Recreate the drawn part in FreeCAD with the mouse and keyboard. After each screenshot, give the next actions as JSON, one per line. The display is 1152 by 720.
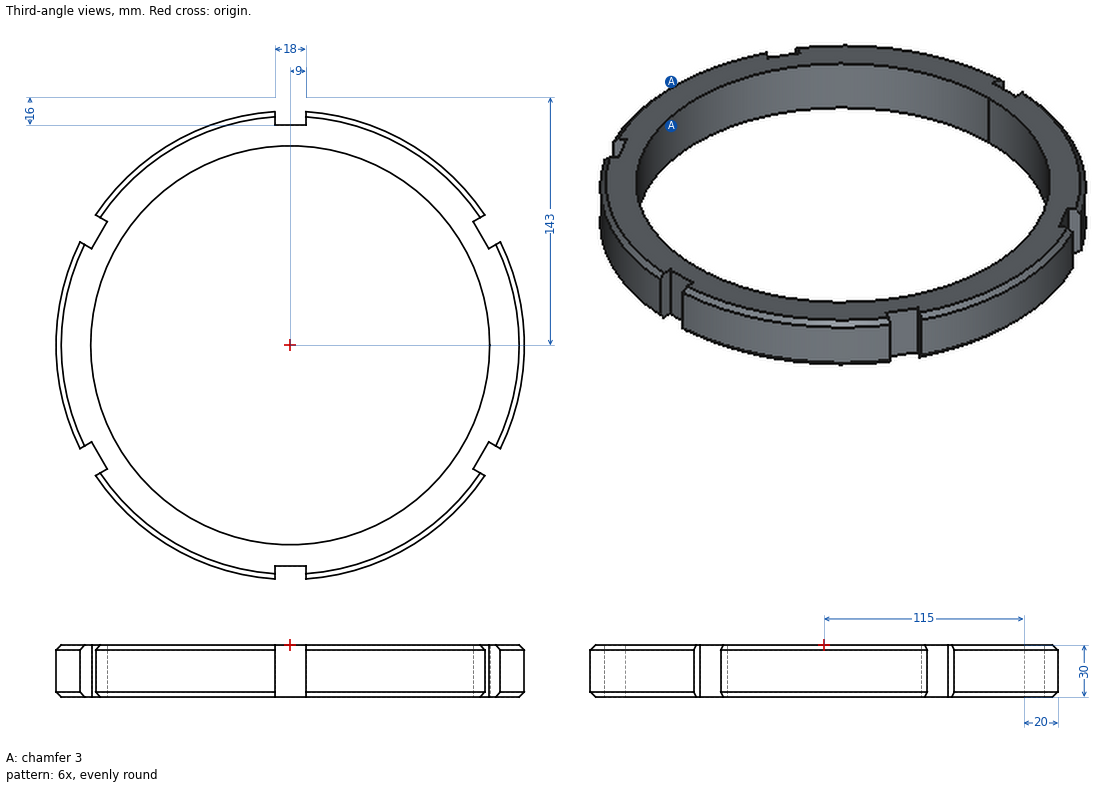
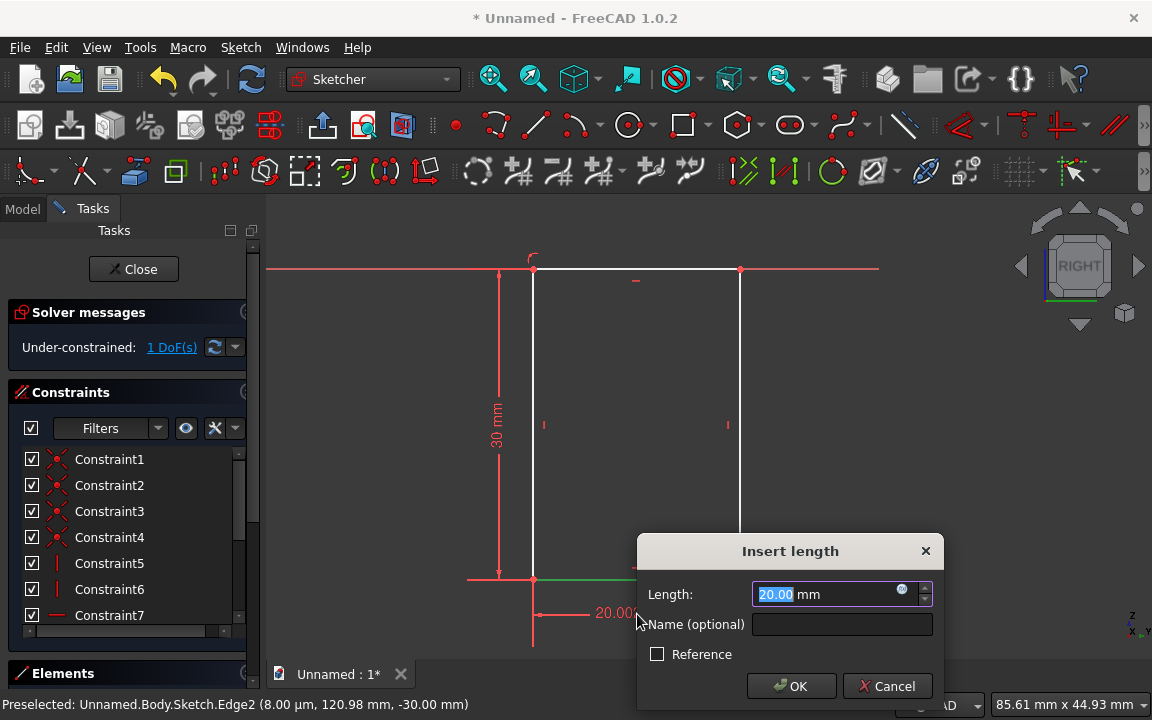
{"action": "type", "text": "20"}
{"action": "key", "text": "Return"}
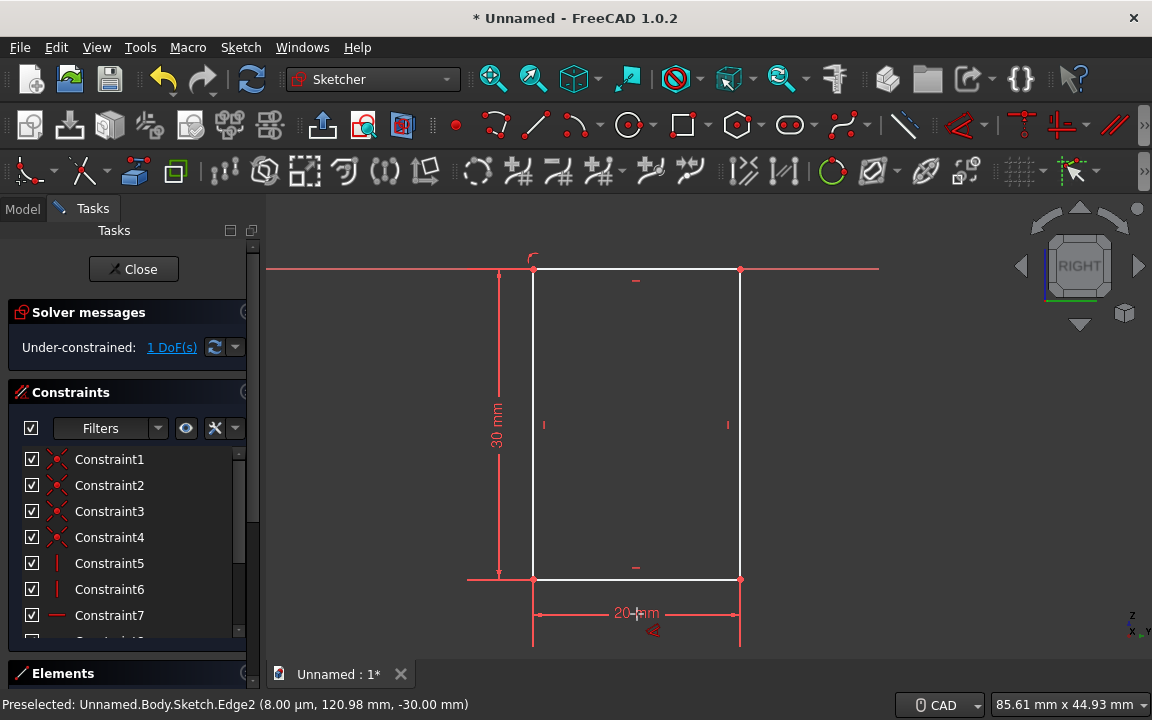
{"action": "left_click", "coordinate": [533, 269]}
{"action": "left_click", "coordinate": [414, 235]}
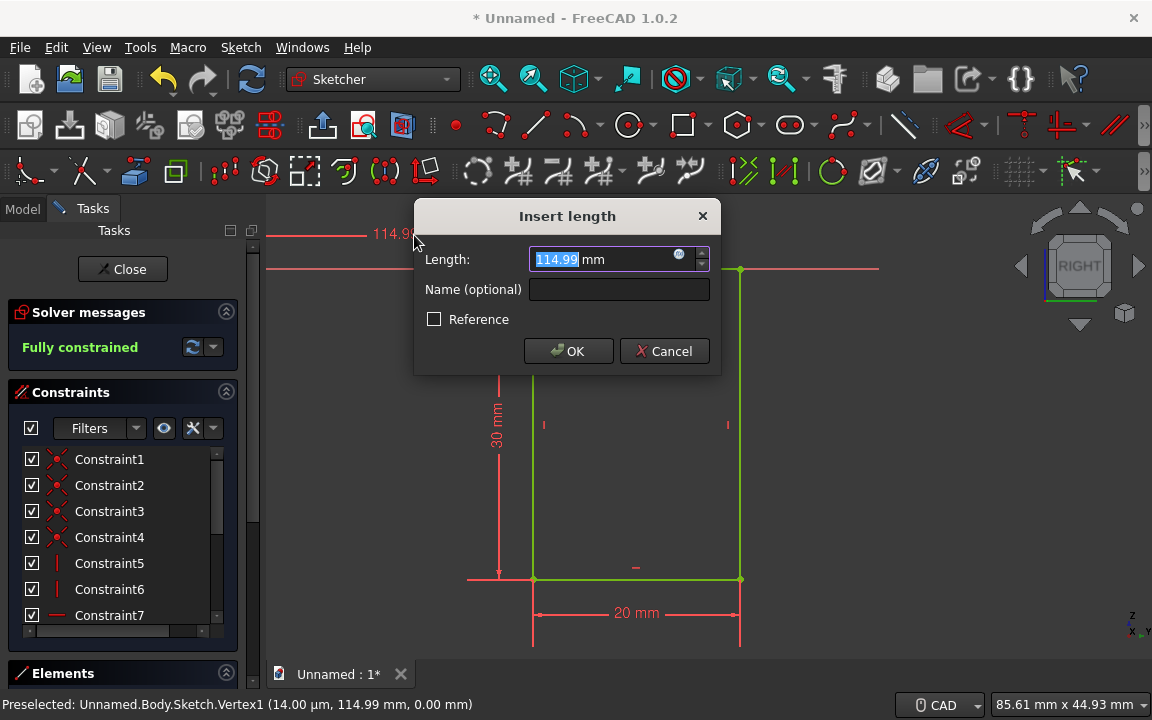
{"action": "type", "text": "115"}
{"action": "key", "text": "Return"}
{"action": "key", "text": "Escape"}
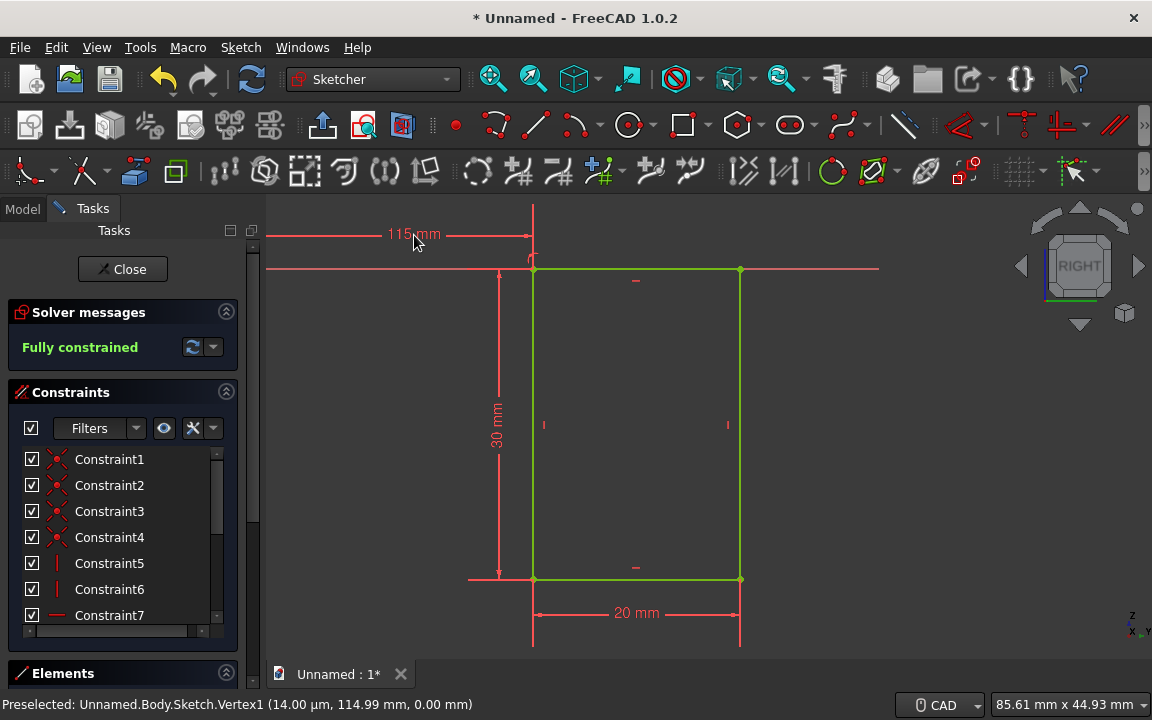
{"action": "left_click", "coordinate": [123, 269]}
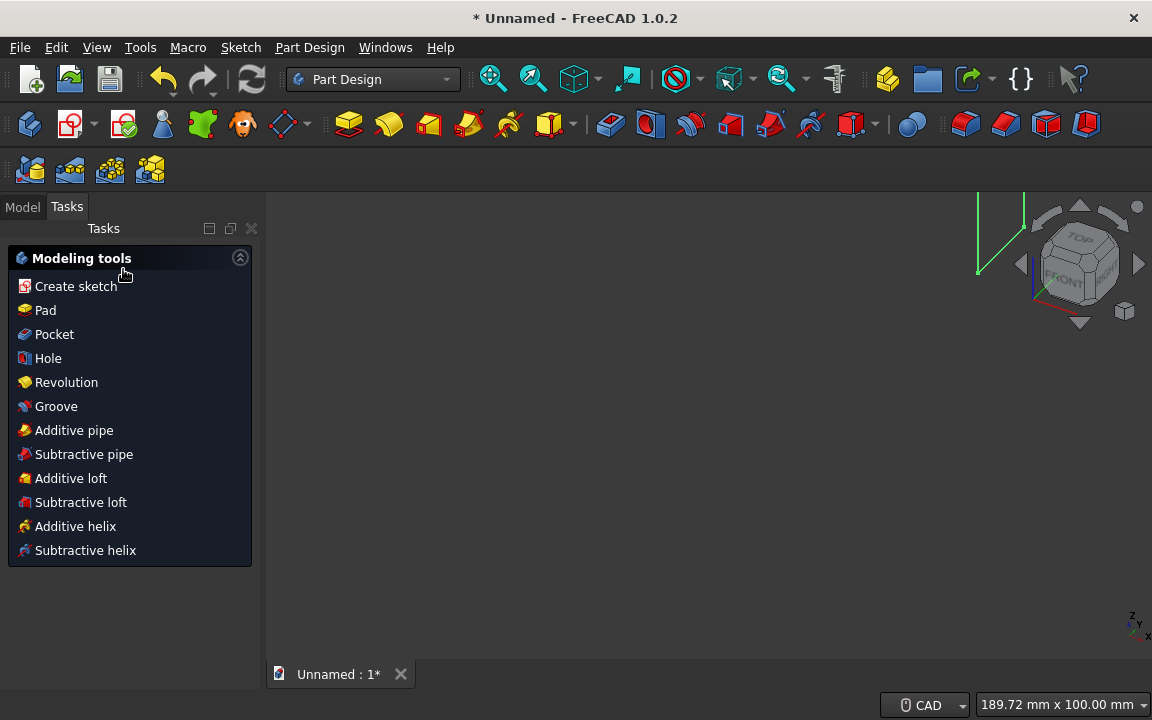
{"action": "left_click", "coordinate": [390, 124]}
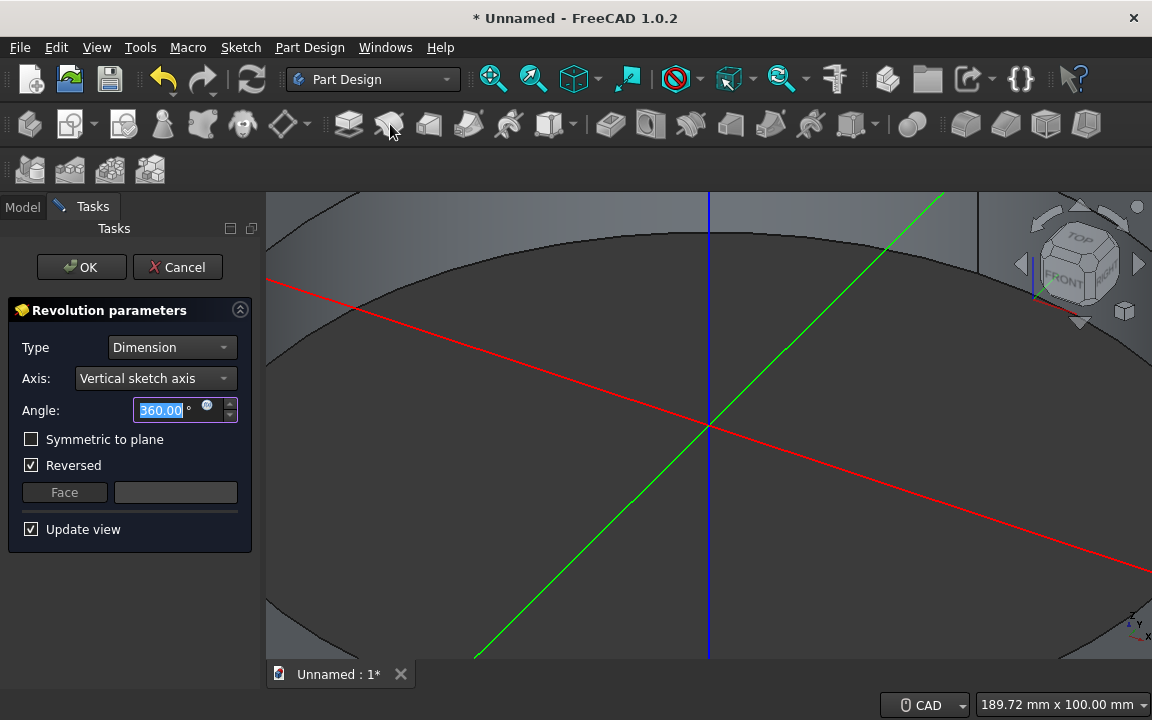
{"action": "left_click", "coordinate": [82, 267]}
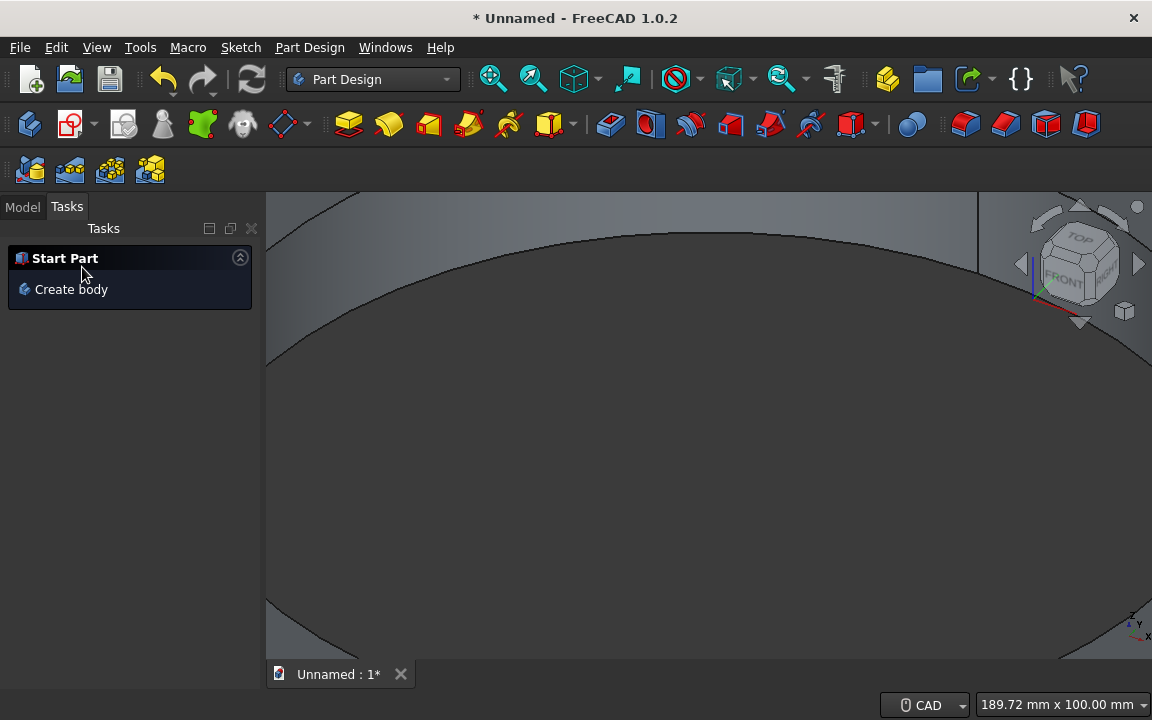
{"action": "left_click", "coordinate": [494, 80]}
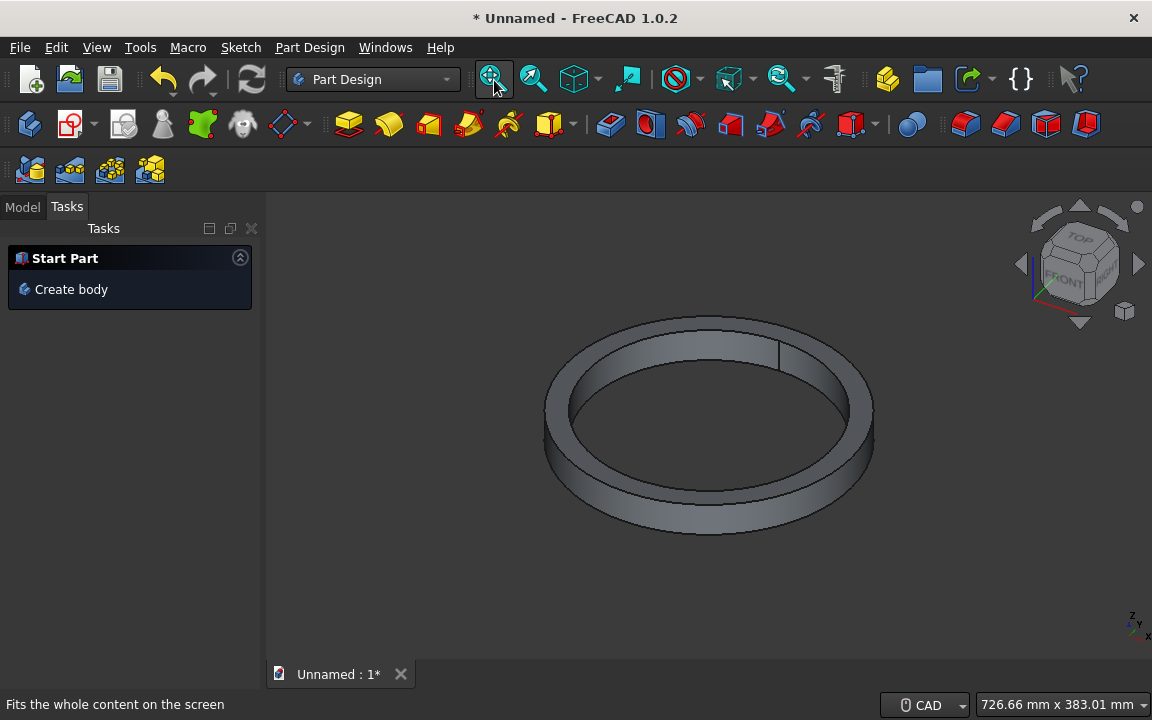
{"action": "left_click", "coordinate": [627, 491]}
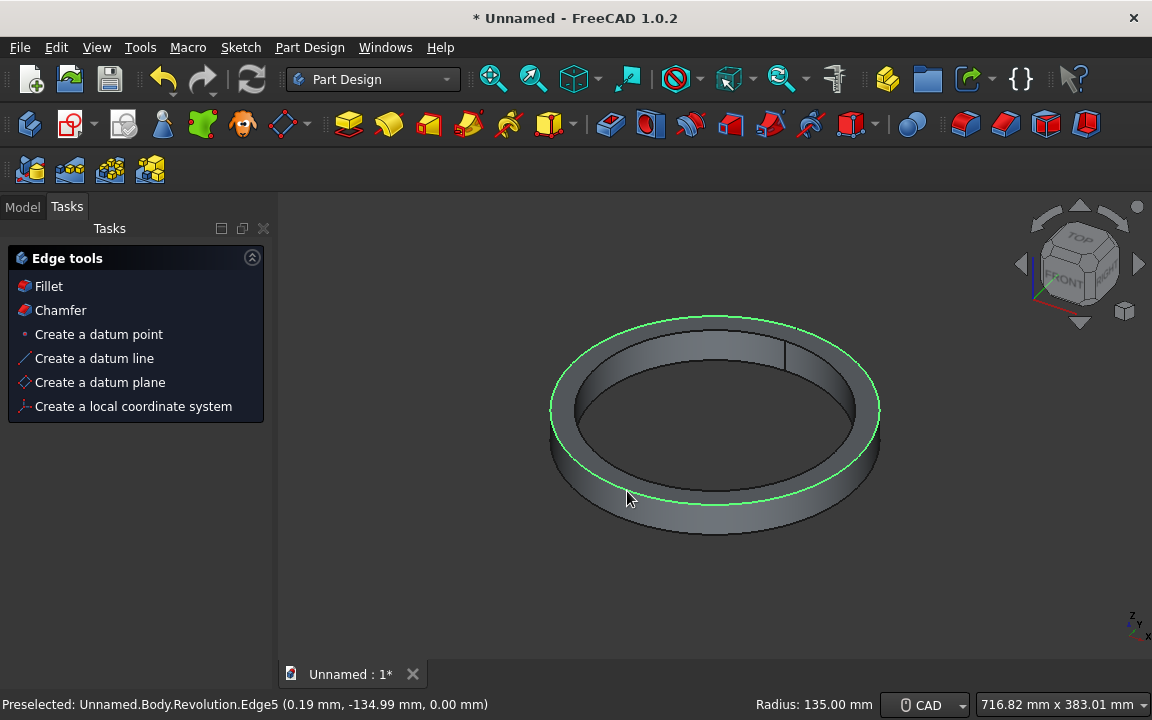
{"action": "key", "text": "0"}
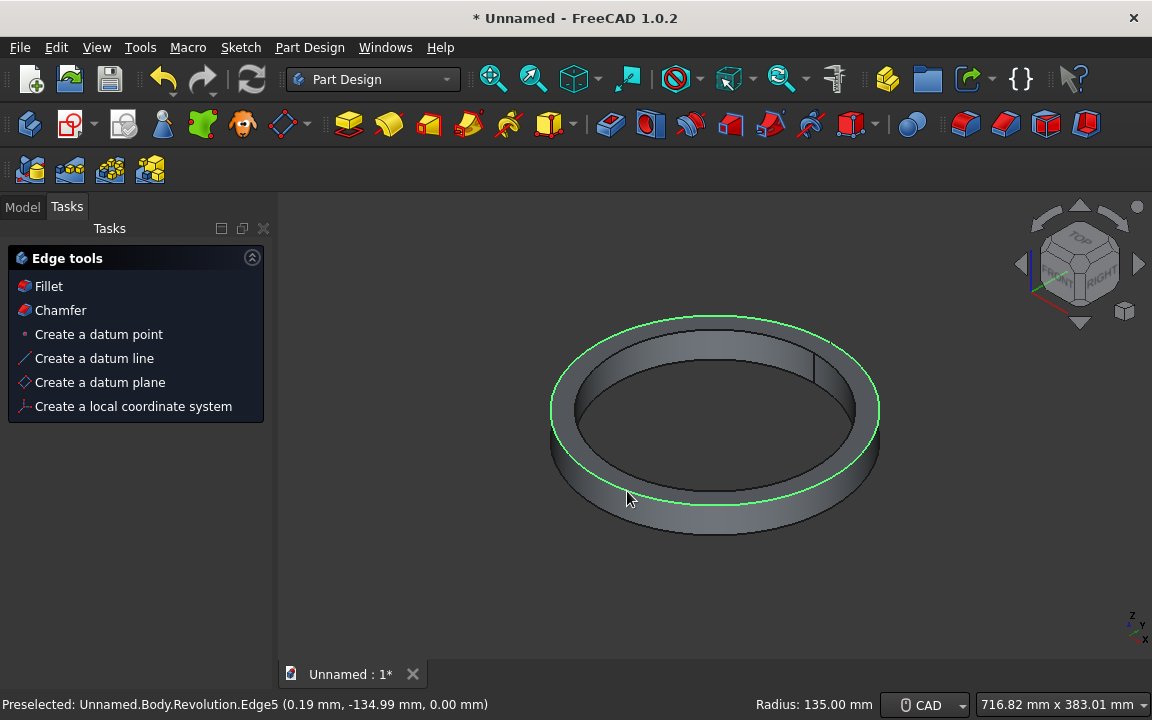
{"action": "key", "text": "2"}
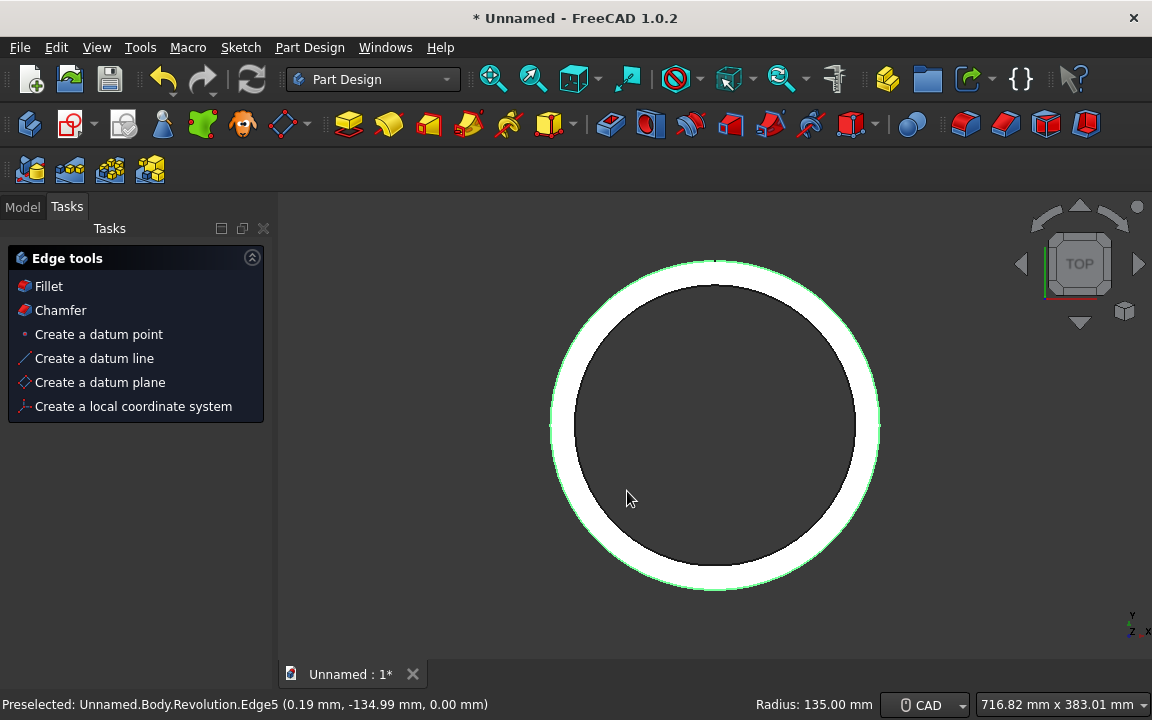
{"action": "key", "text": "1"}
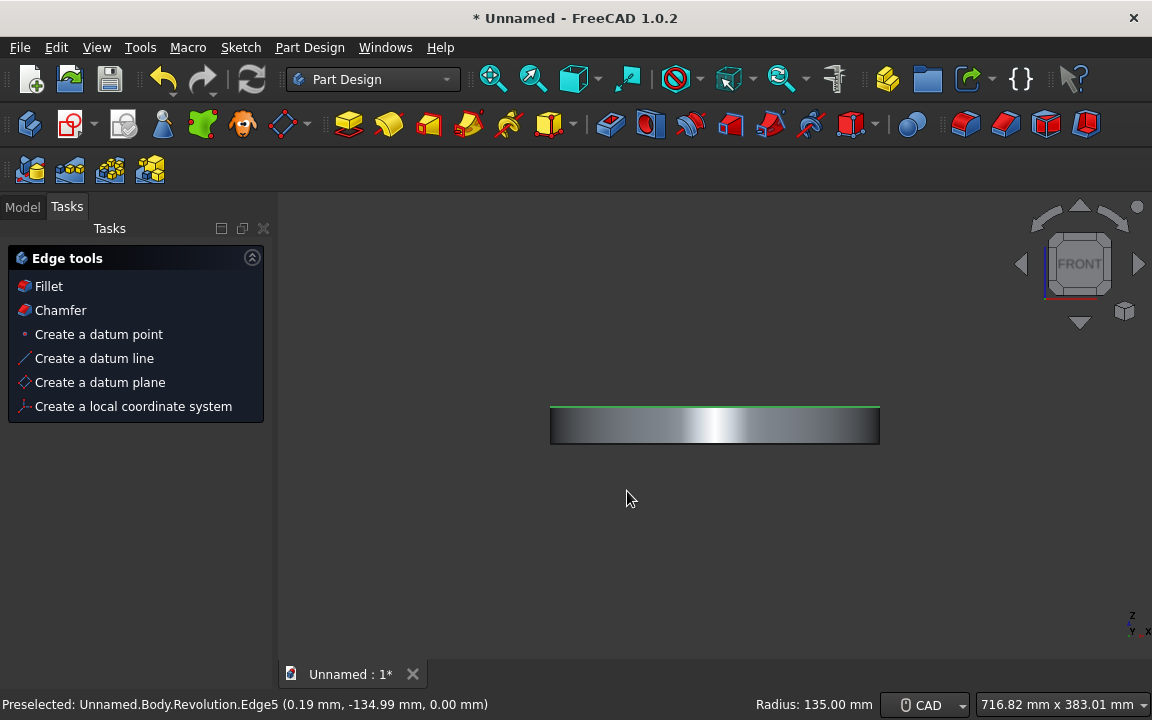
{"action": "left_click", "coordinate": [494, 80]}